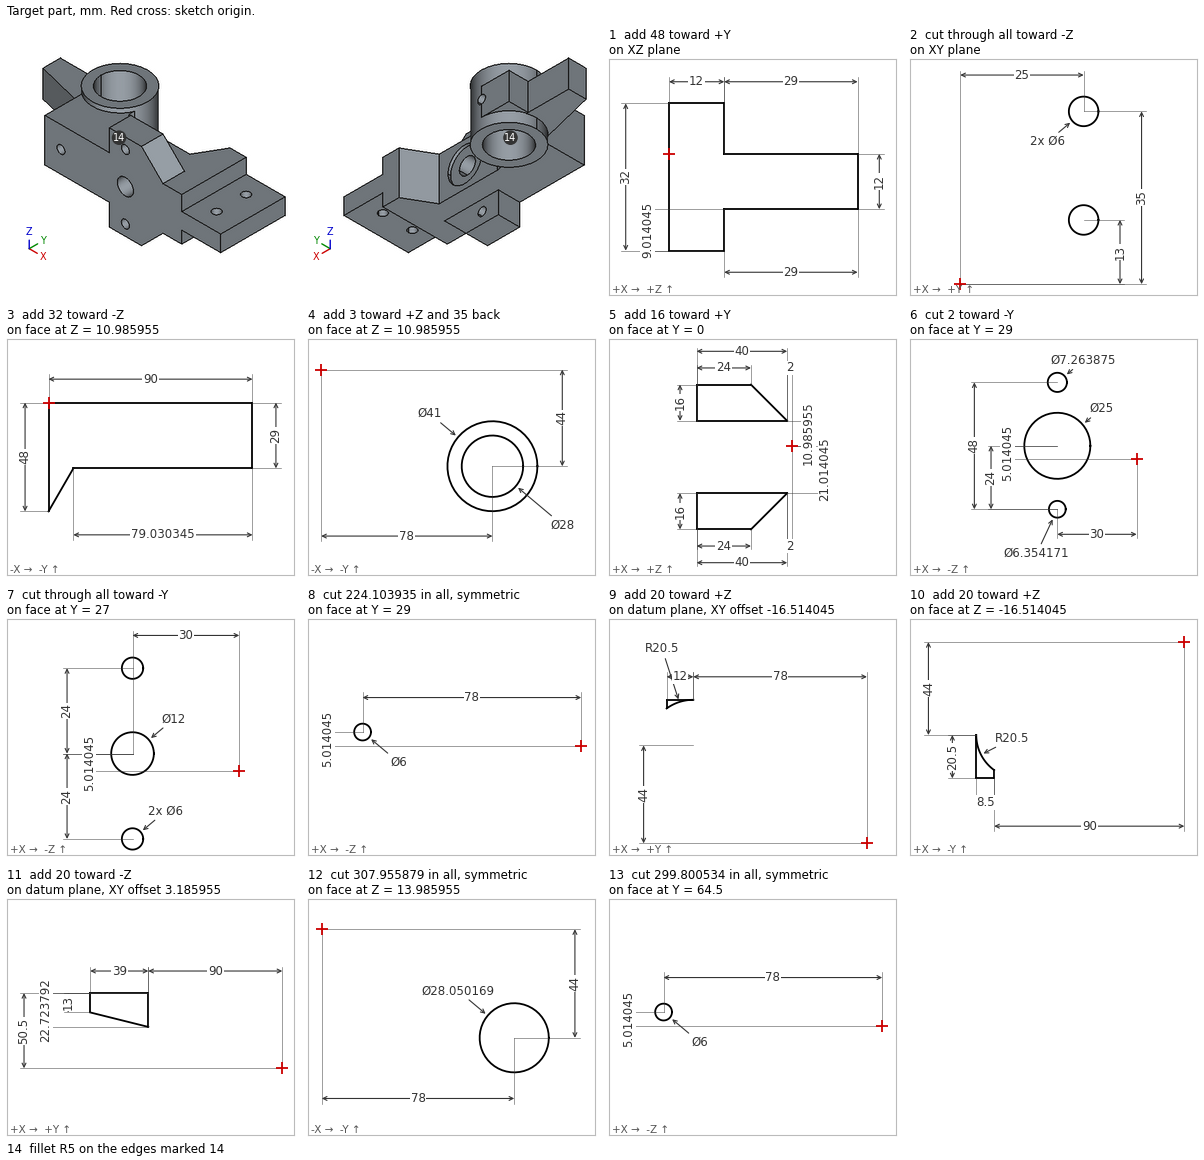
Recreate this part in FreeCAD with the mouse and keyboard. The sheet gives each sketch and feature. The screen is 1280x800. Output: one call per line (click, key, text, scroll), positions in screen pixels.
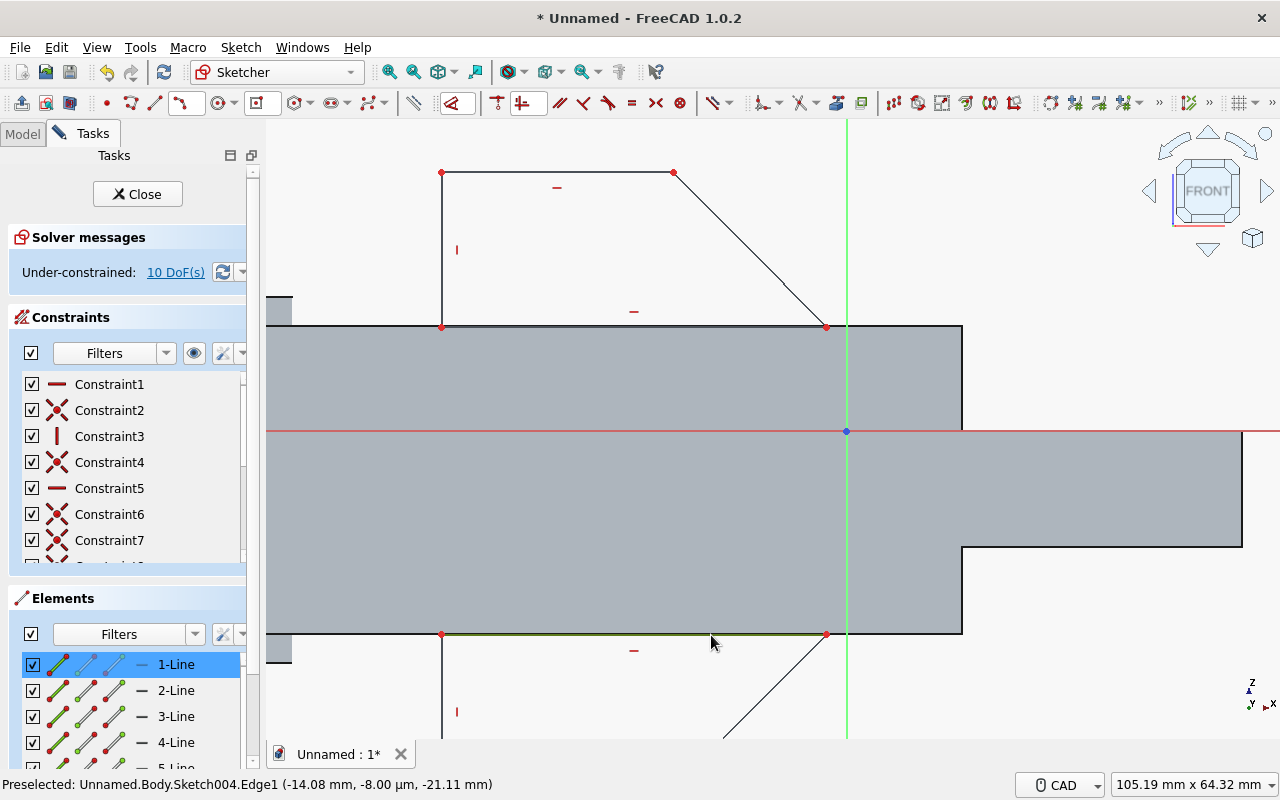
click(470, 104)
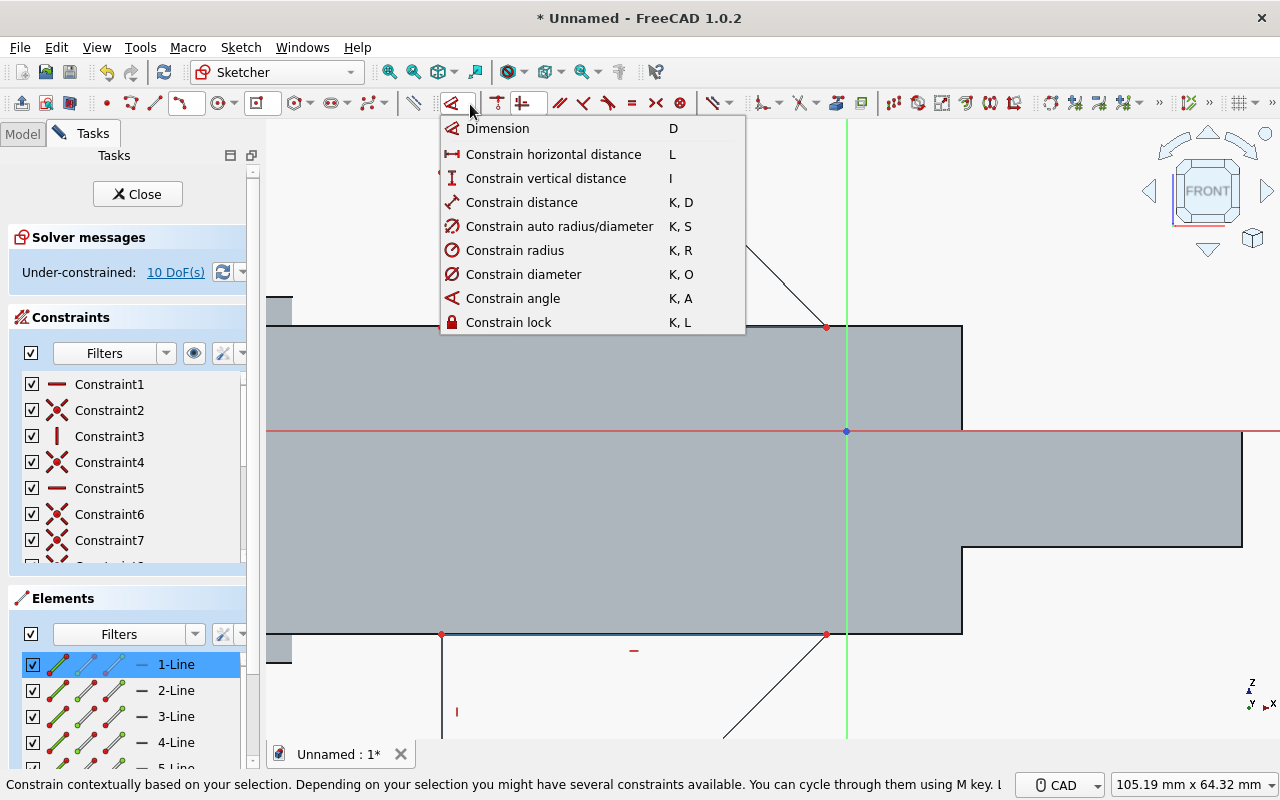
click(593, 154)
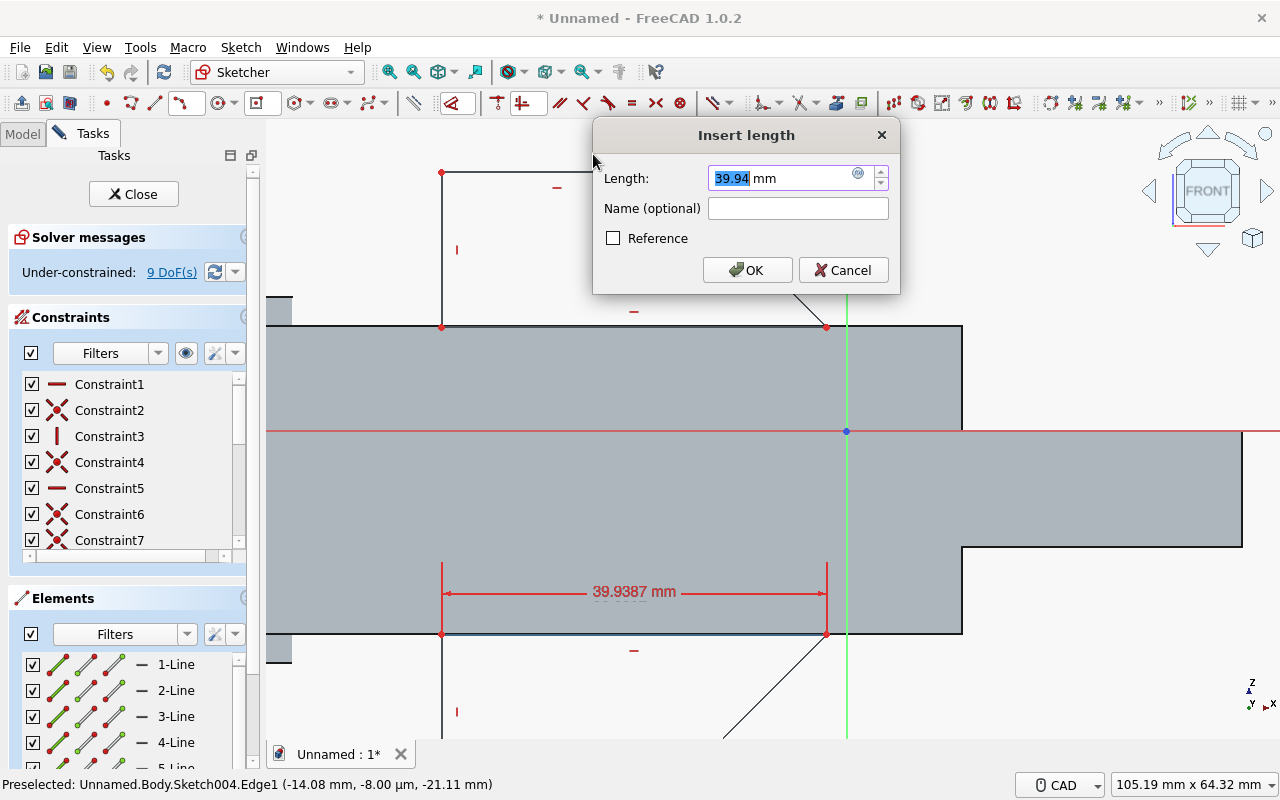
text(40)
key(Return)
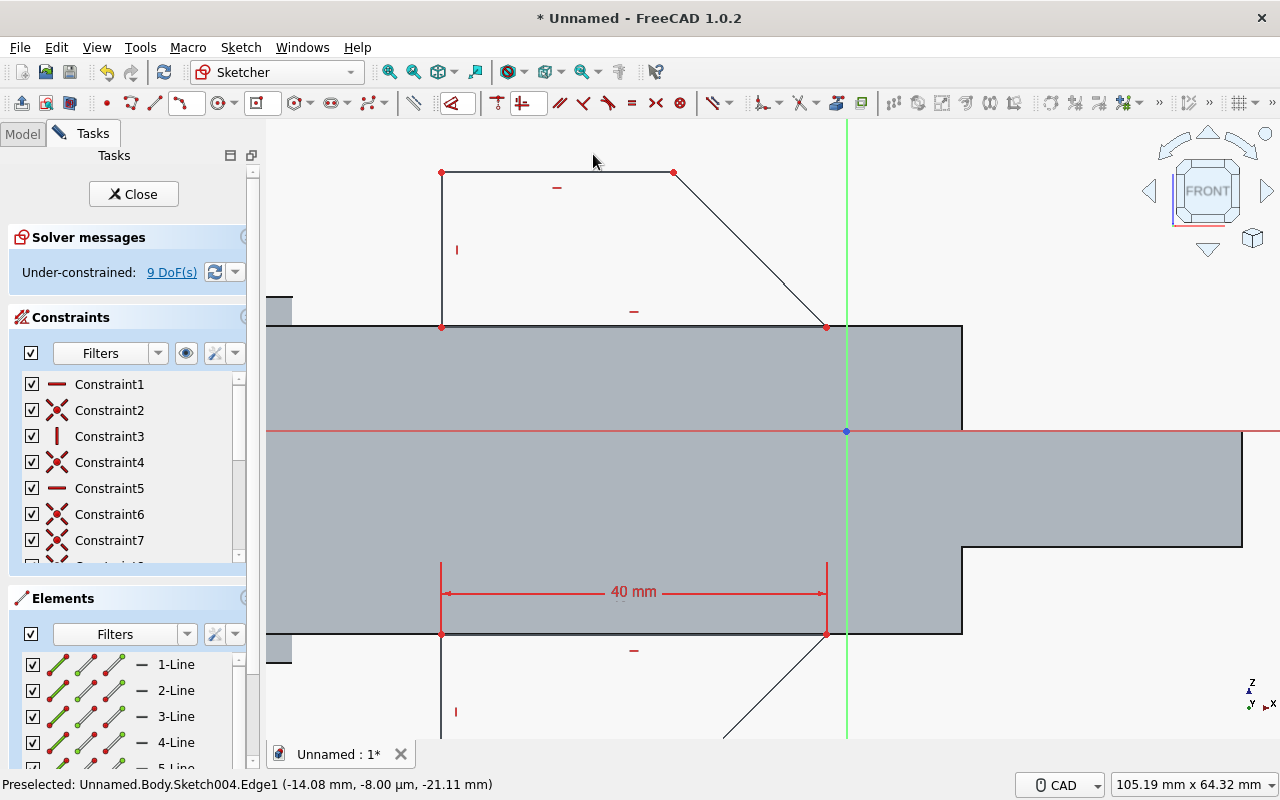
click(441, 681)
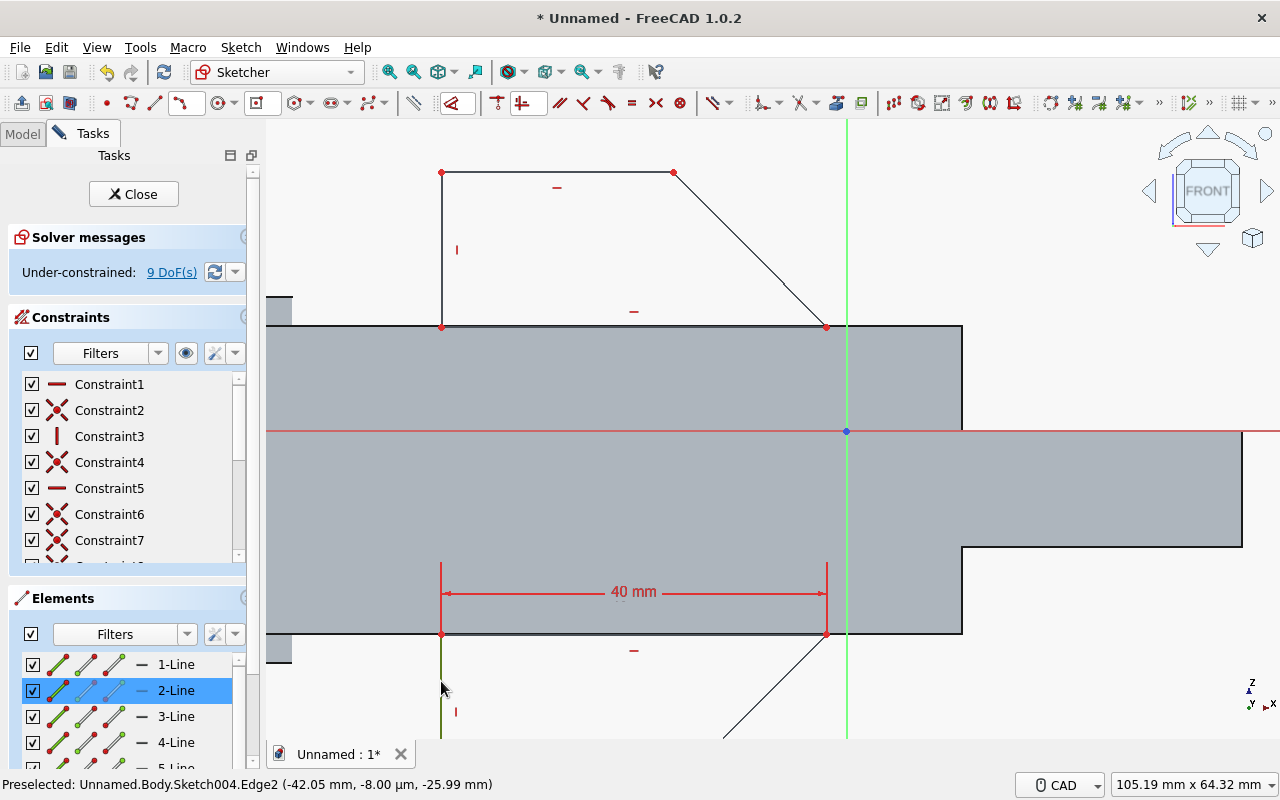
key(i)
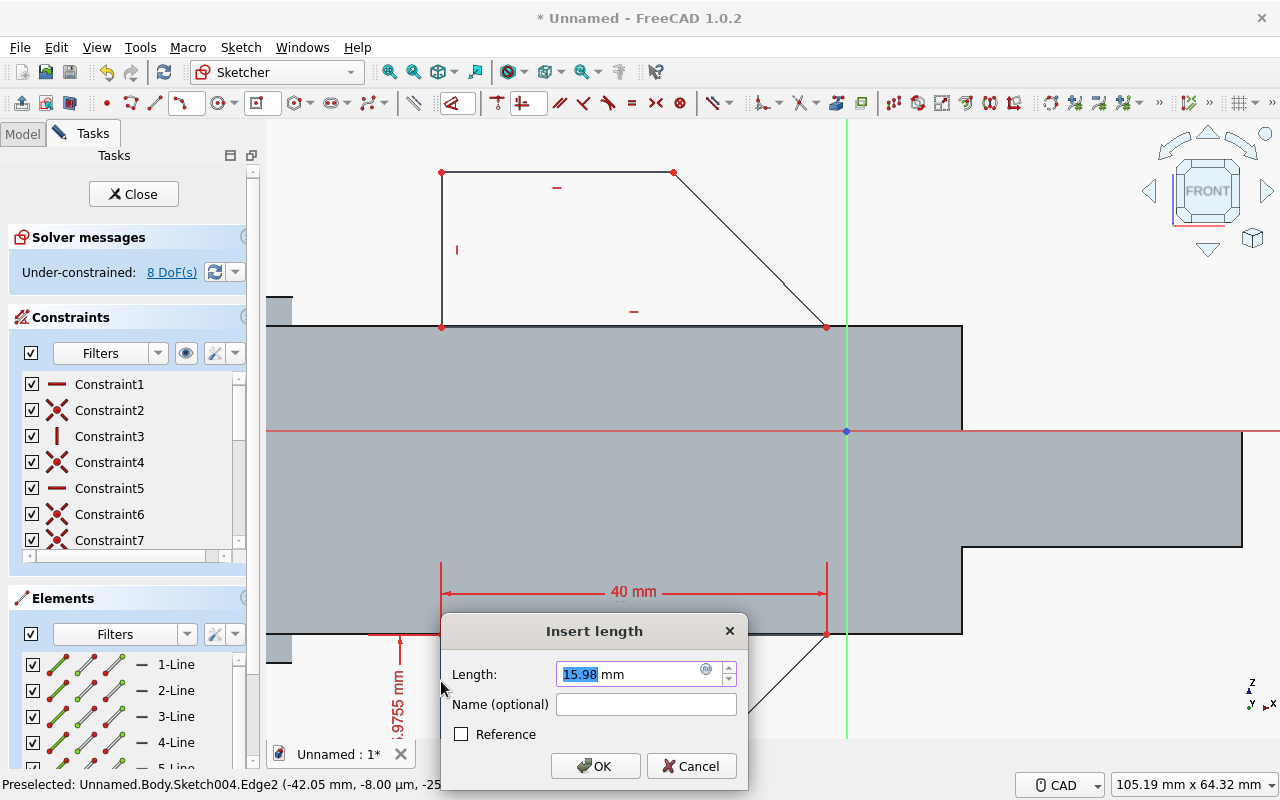
text(16)
key(Return)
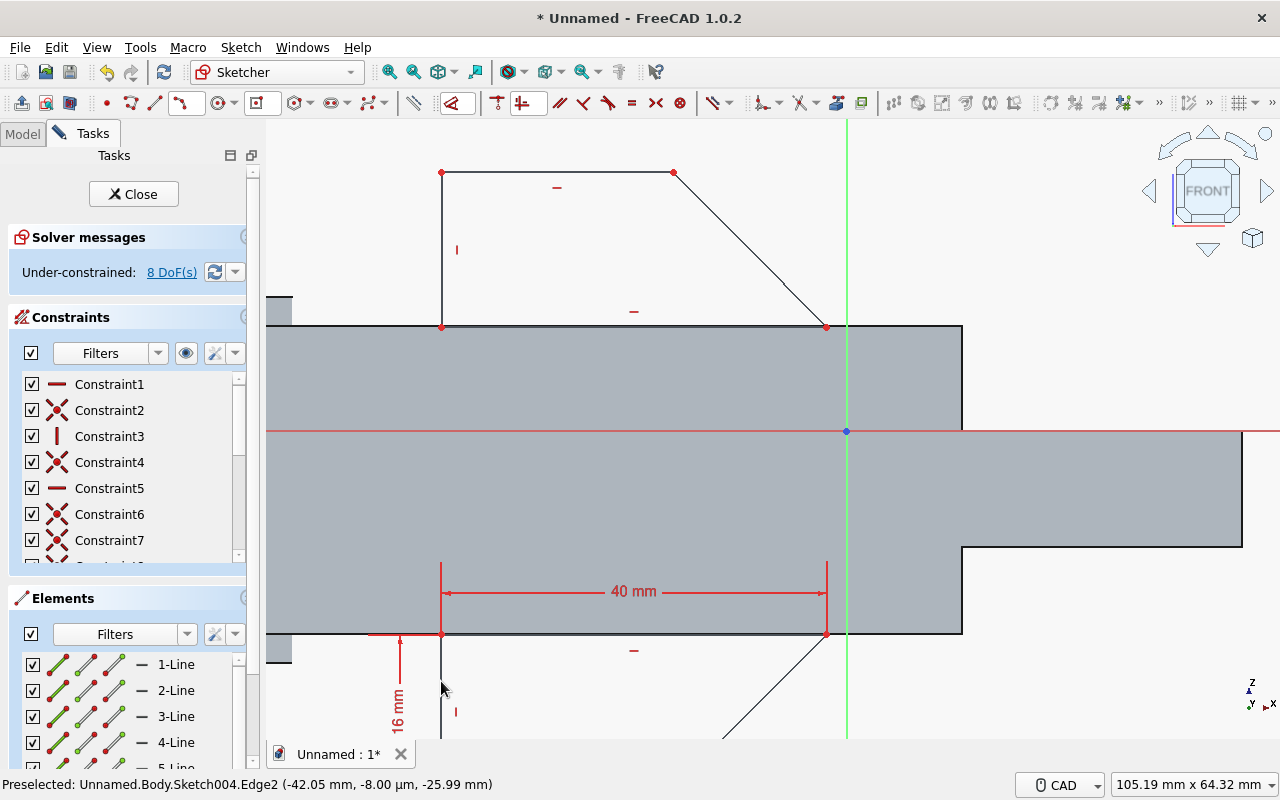
scroll(827, 326, down, 2)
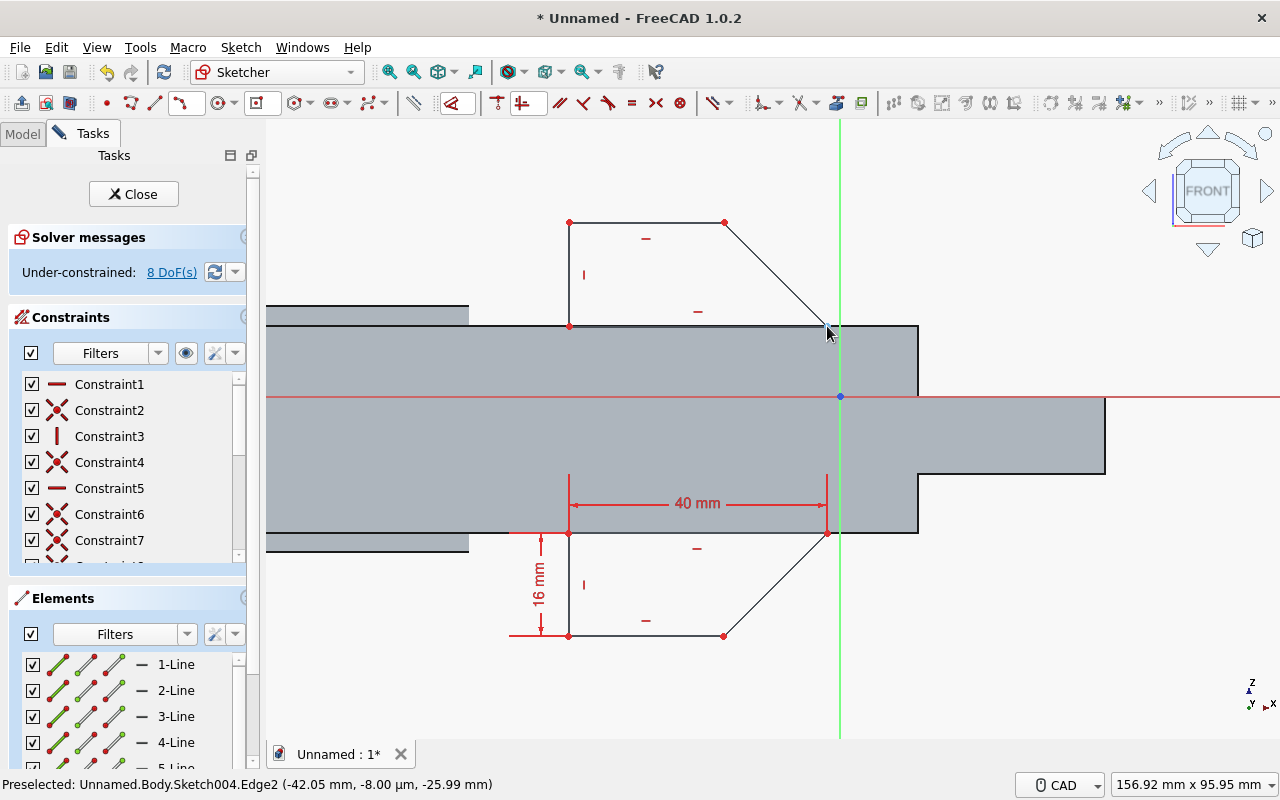
click(615, 636)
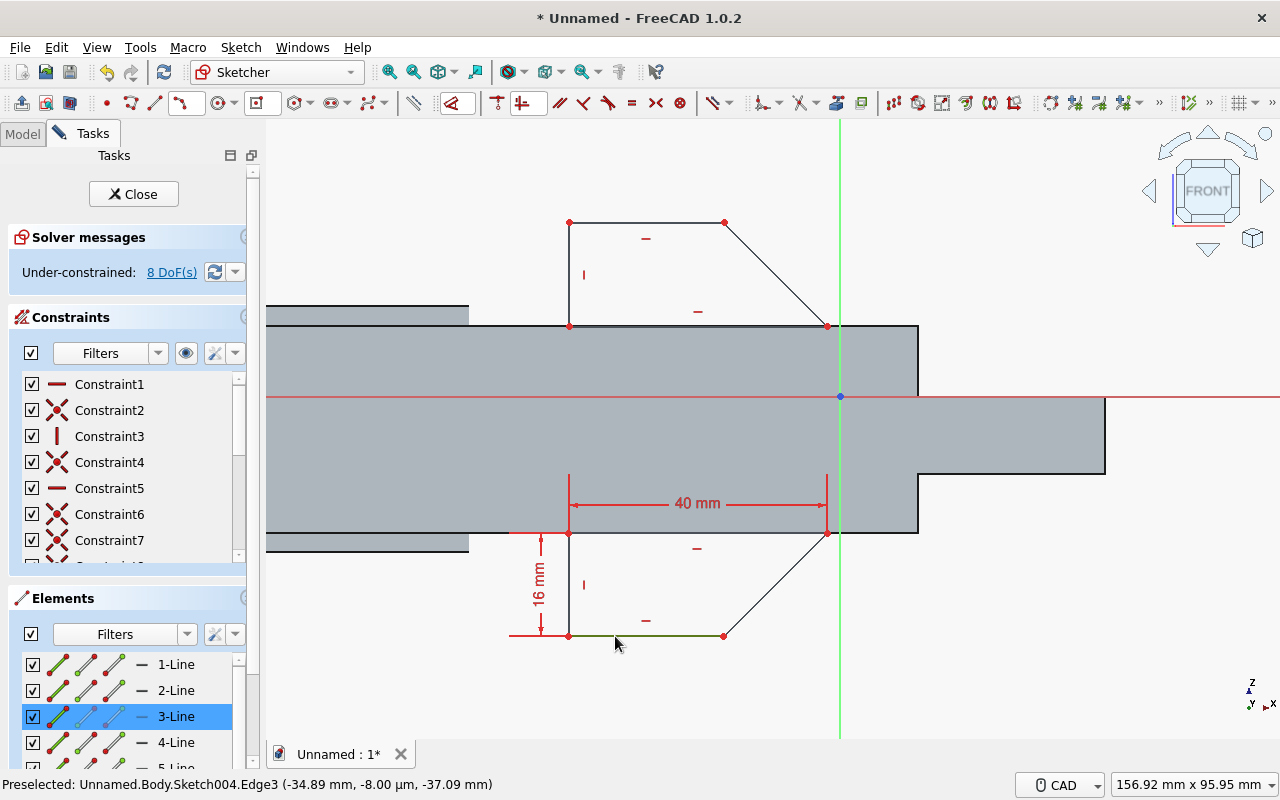
key(l)